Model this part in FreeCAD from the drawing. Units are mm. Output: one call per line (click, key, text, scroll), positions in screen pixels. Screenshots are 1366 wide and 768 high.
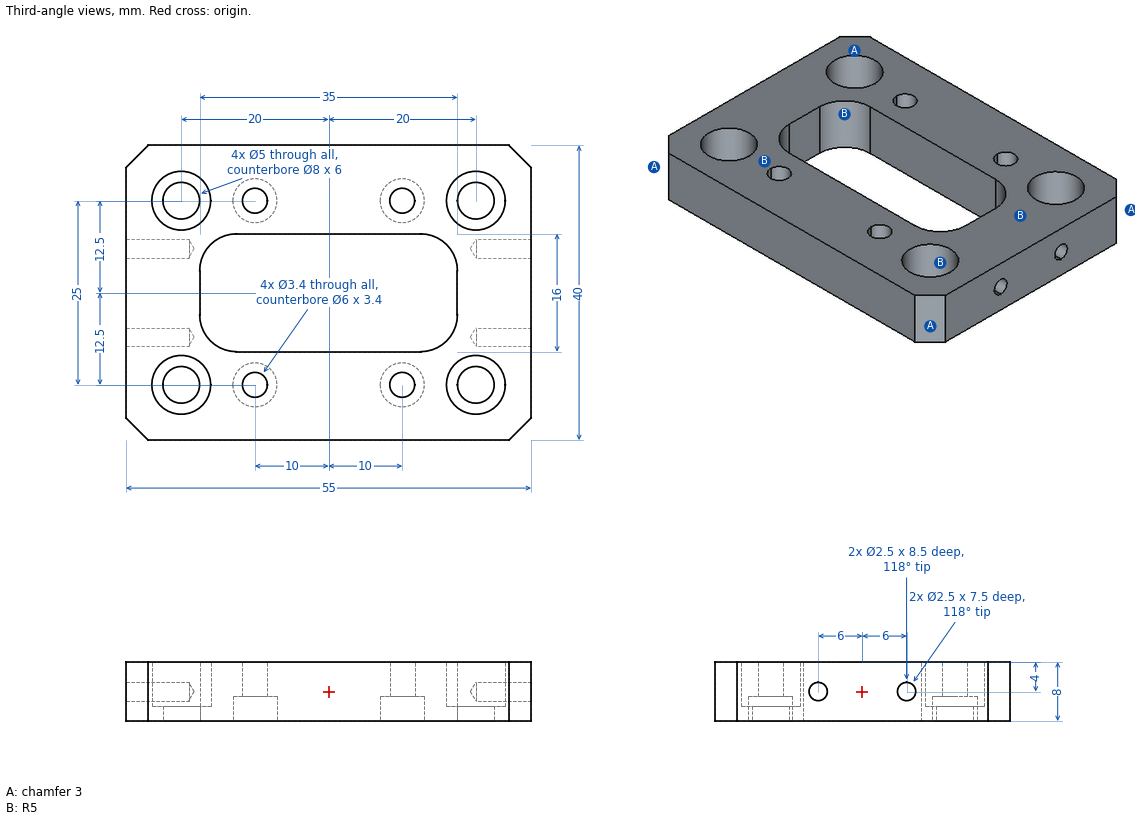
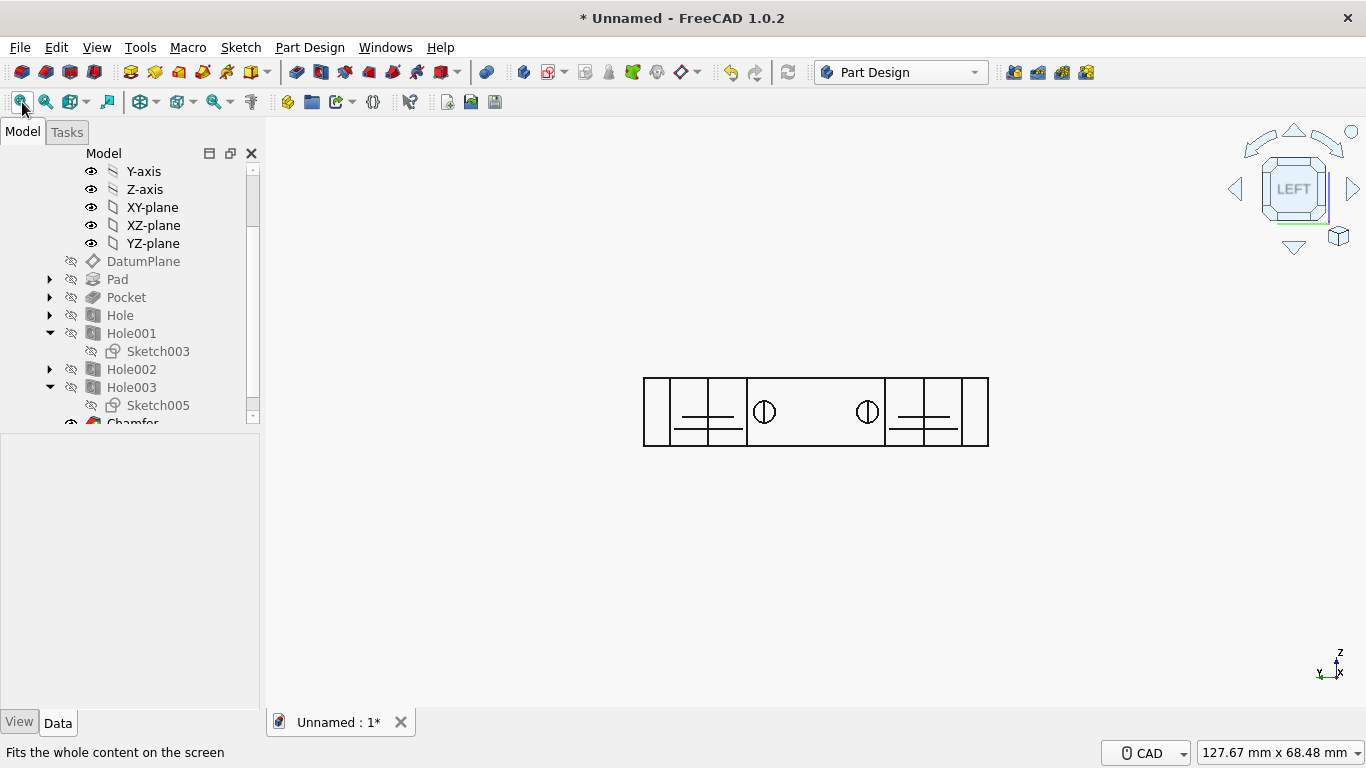
key(0)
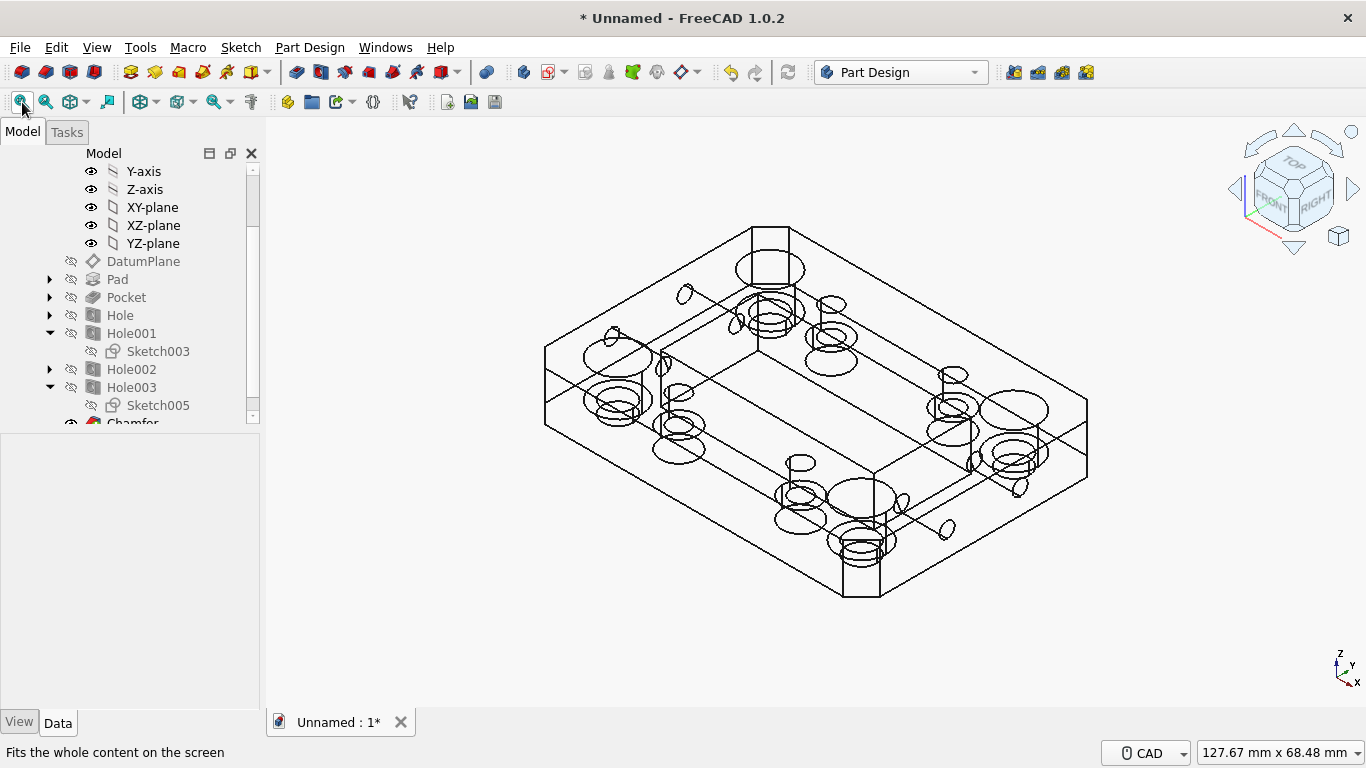
click(661, 378)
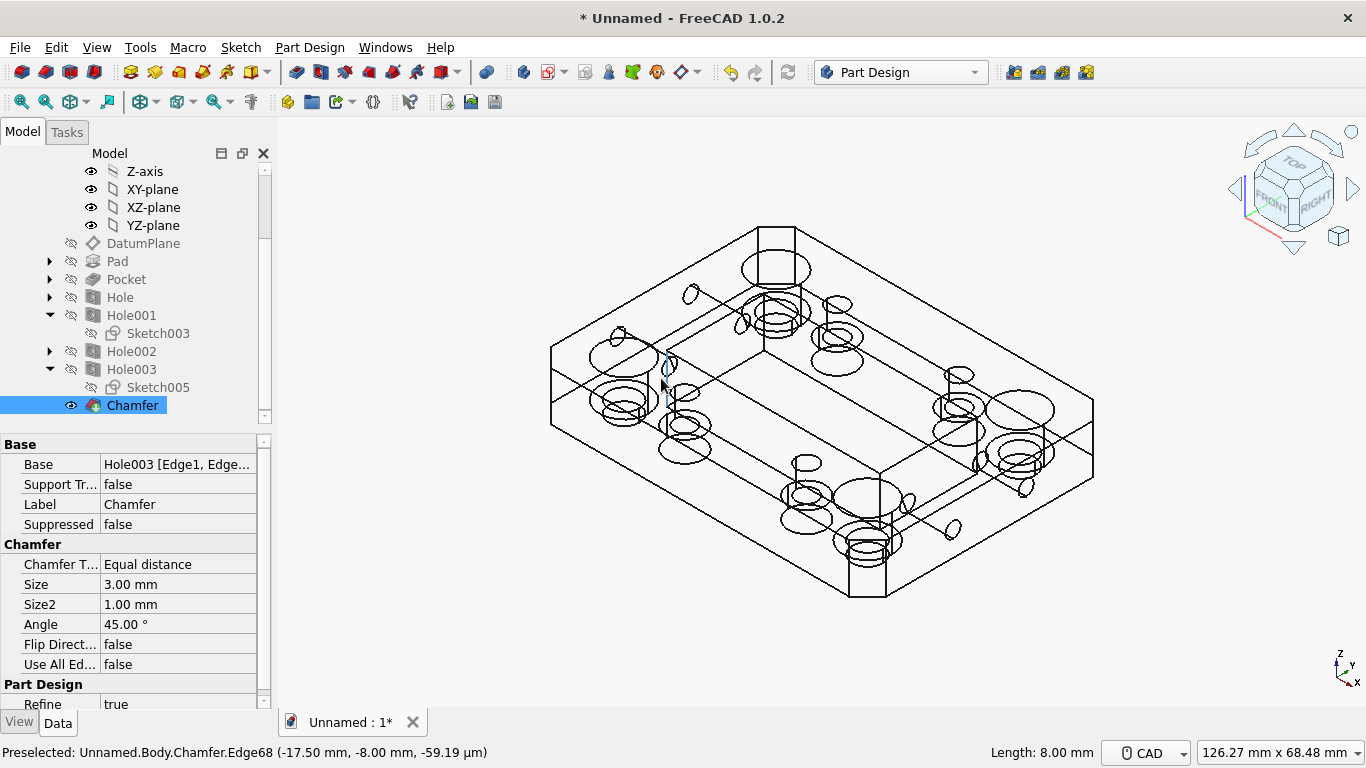
click(880, 501, ctrl)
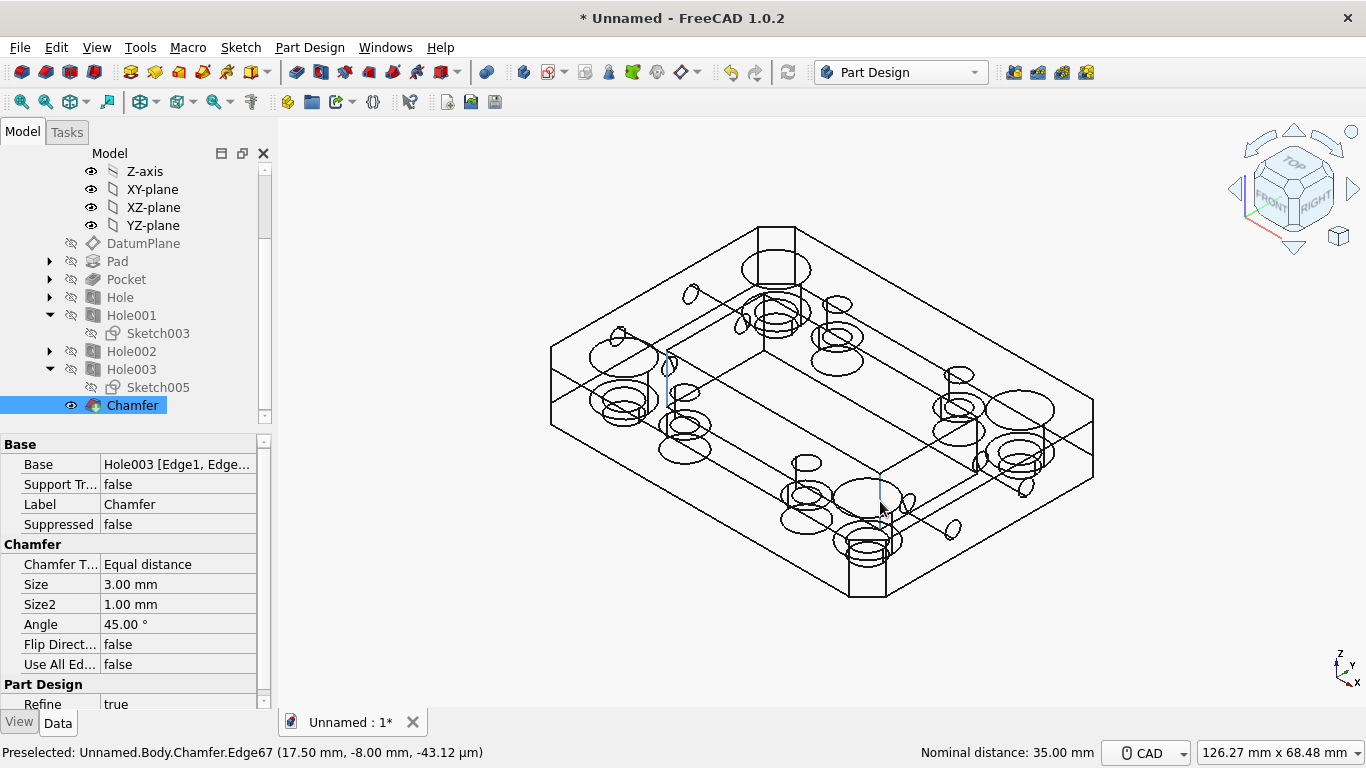
click(977, 444, ctrl)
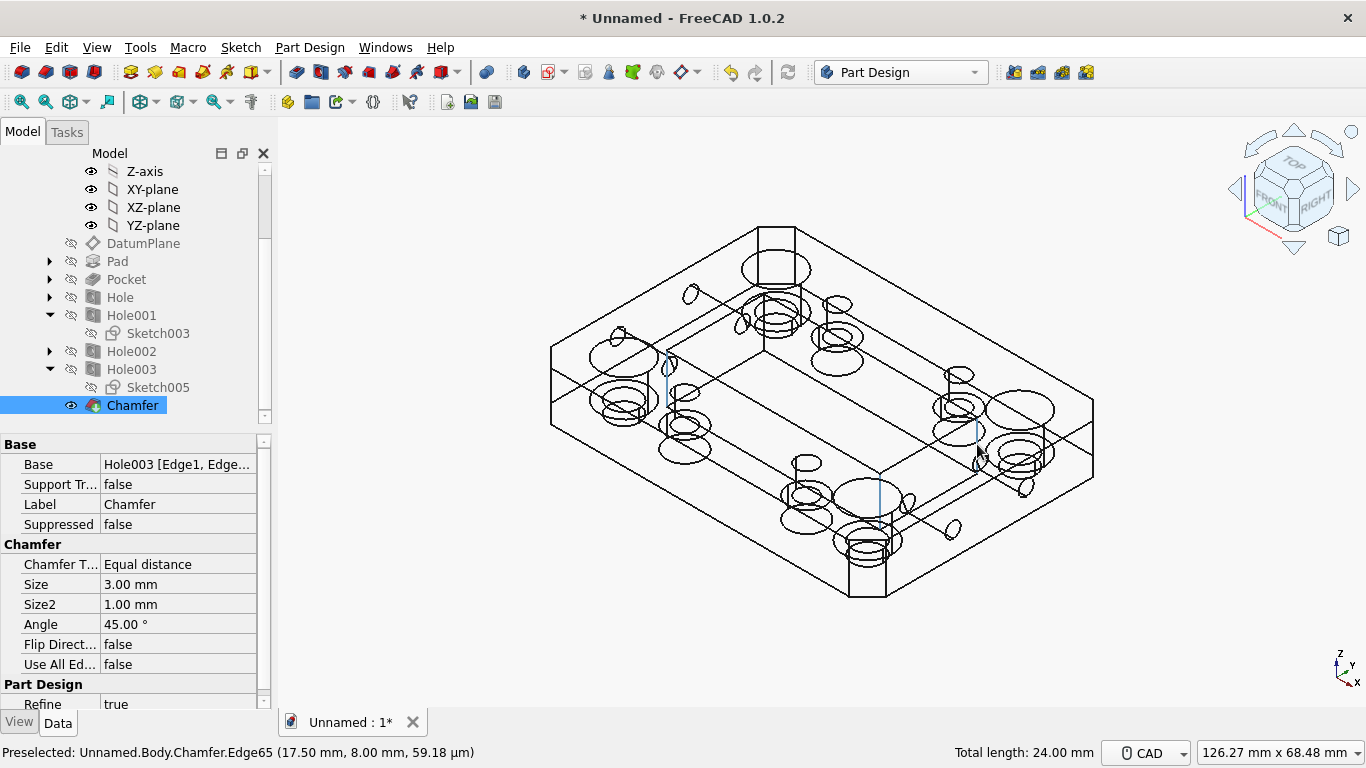
click(764, 321, ctrl)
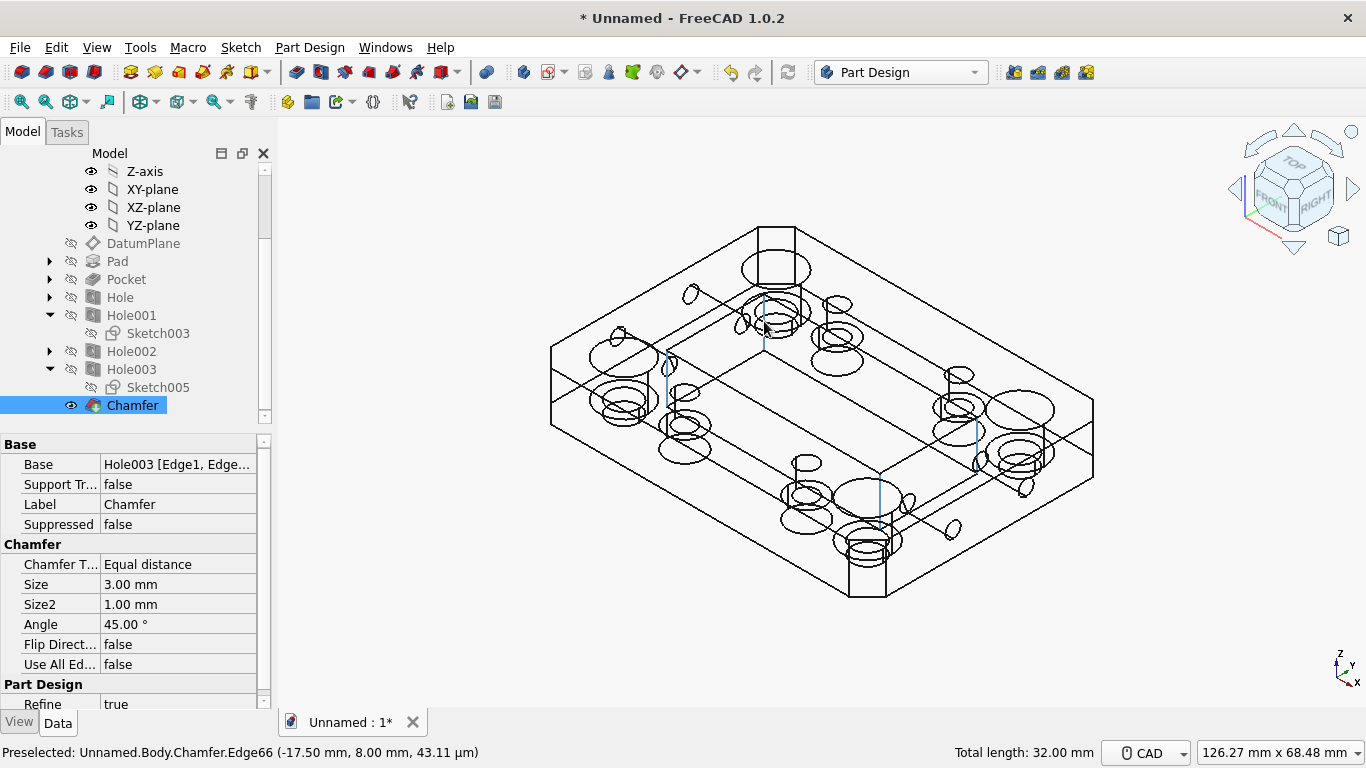
key(v)
key(1)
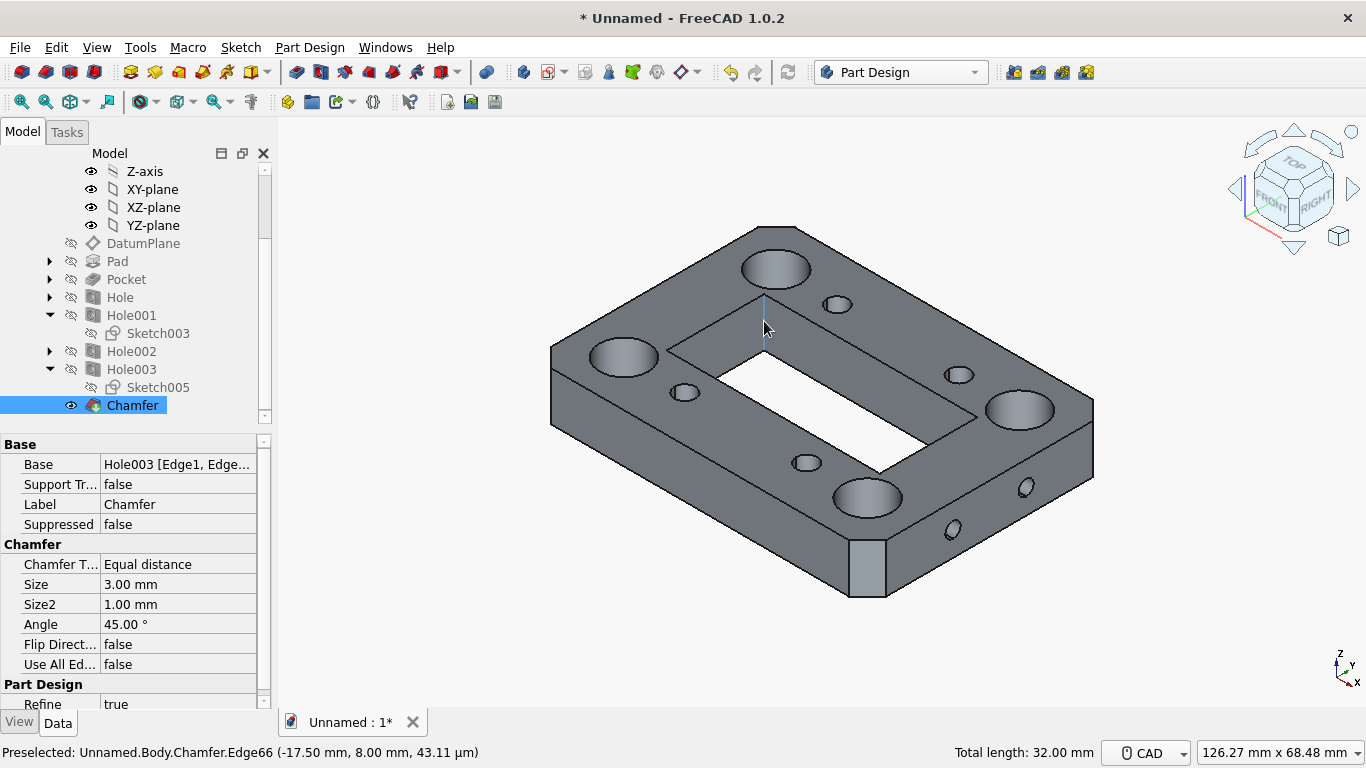
click(22, 72)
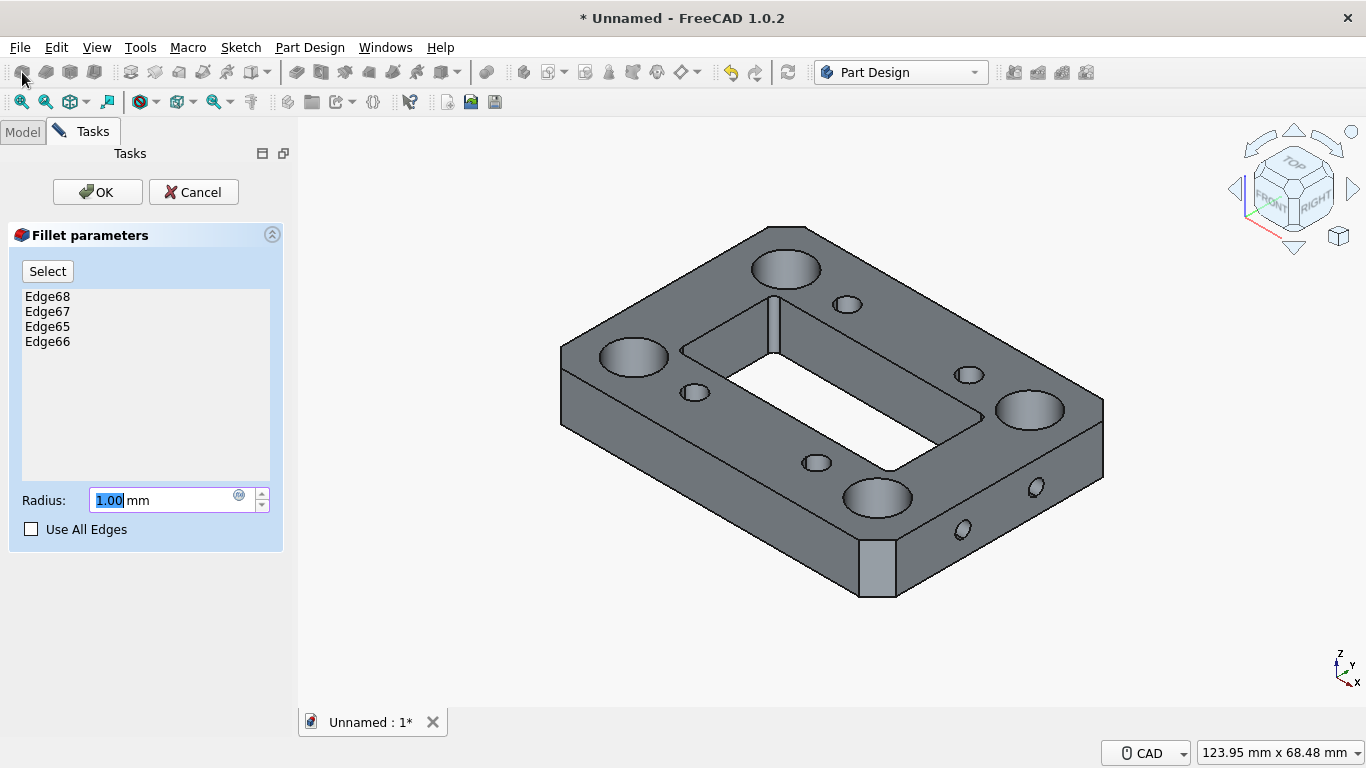
text(5)
key(Tab)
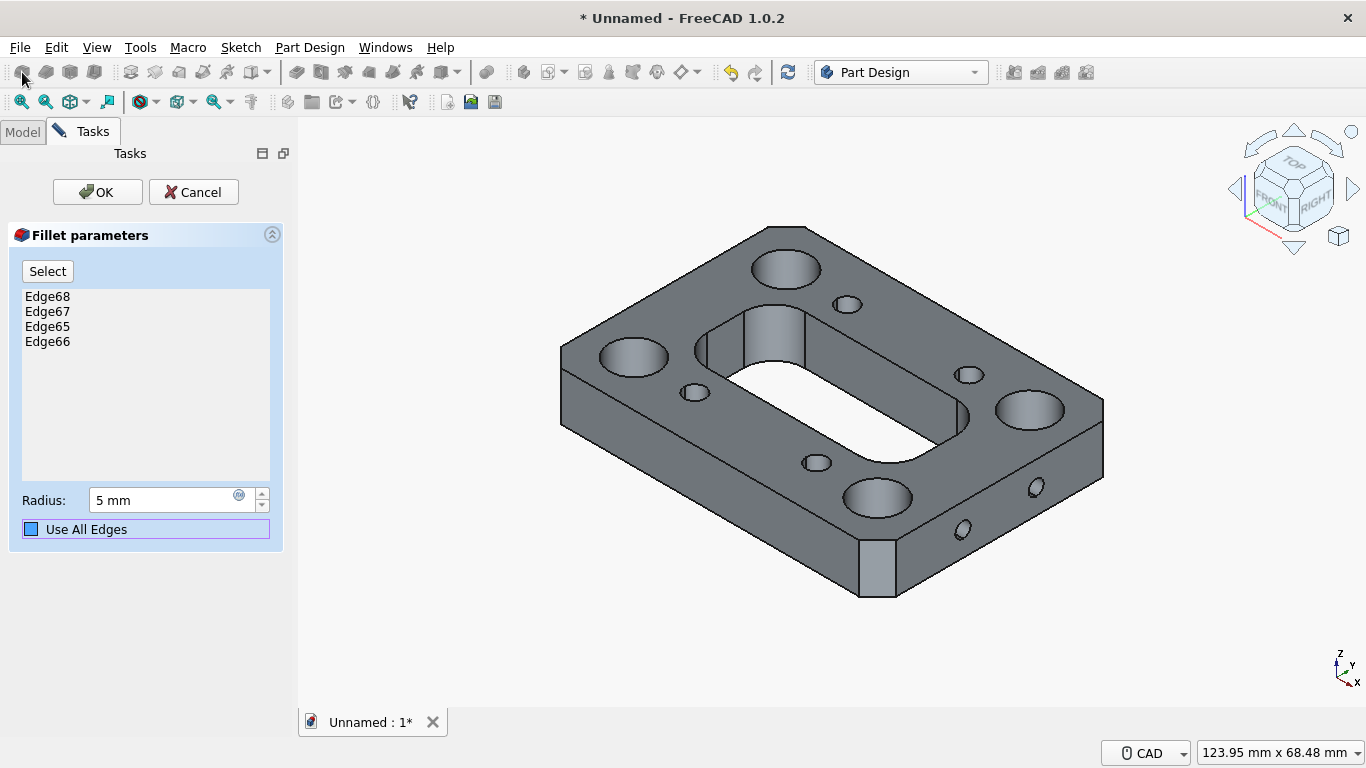
click(98, 192)